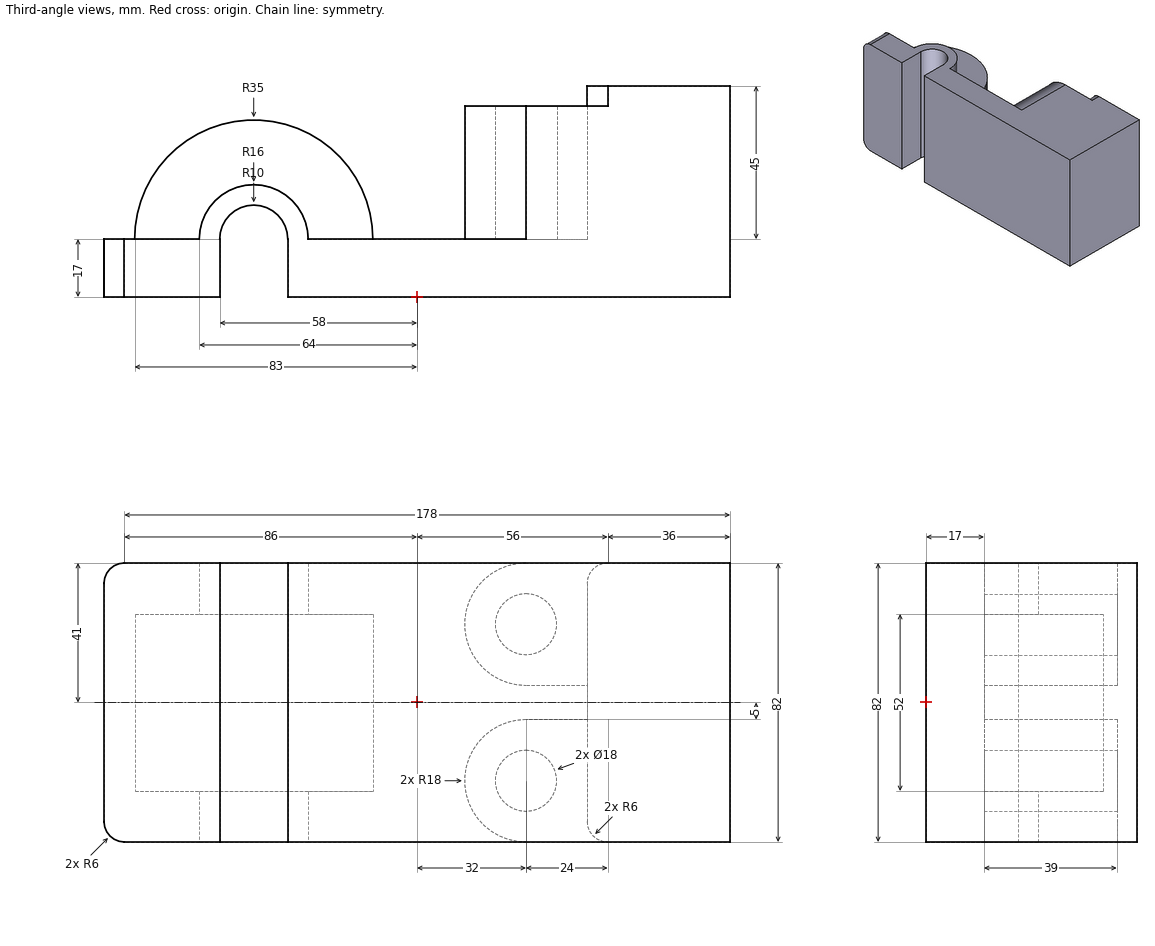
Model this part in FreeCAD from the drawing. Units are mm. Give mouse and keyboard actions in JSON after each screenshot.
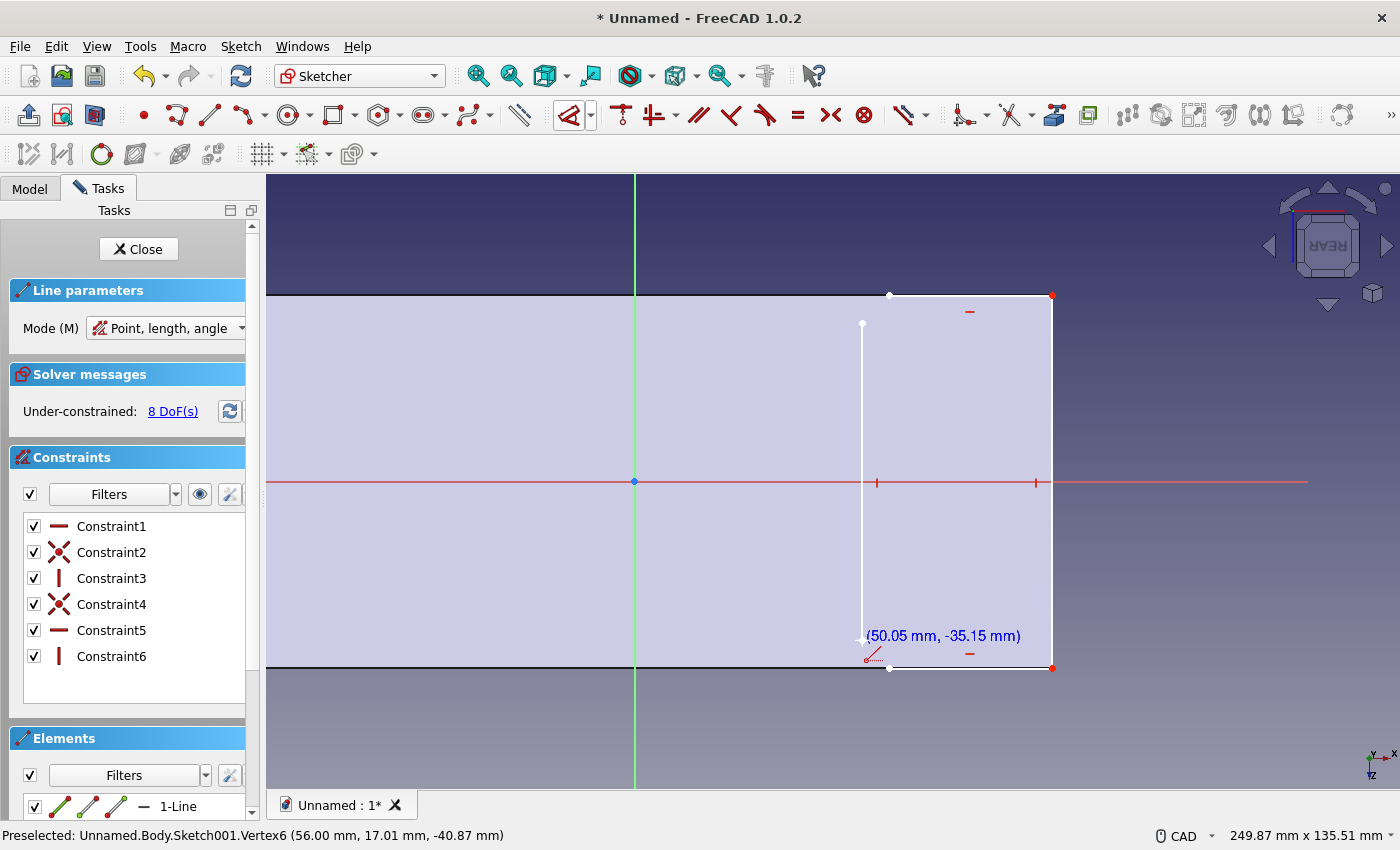
{"action": "left_click", "coordinate": [242, 116]}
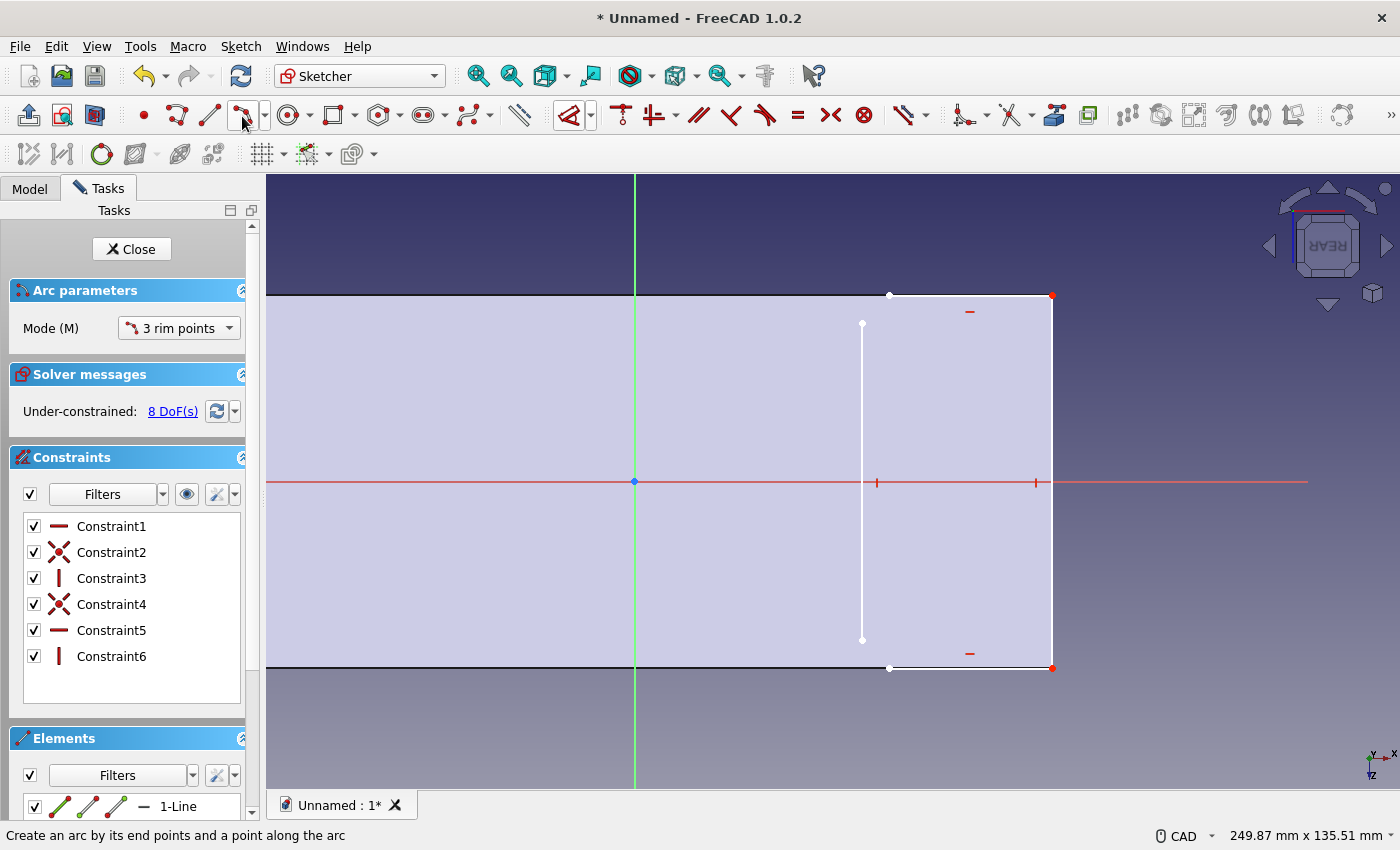
{"action": "left_click", "coordinate": [889, 296]}
{"action": "left_click", "coordinate": [862, 324]}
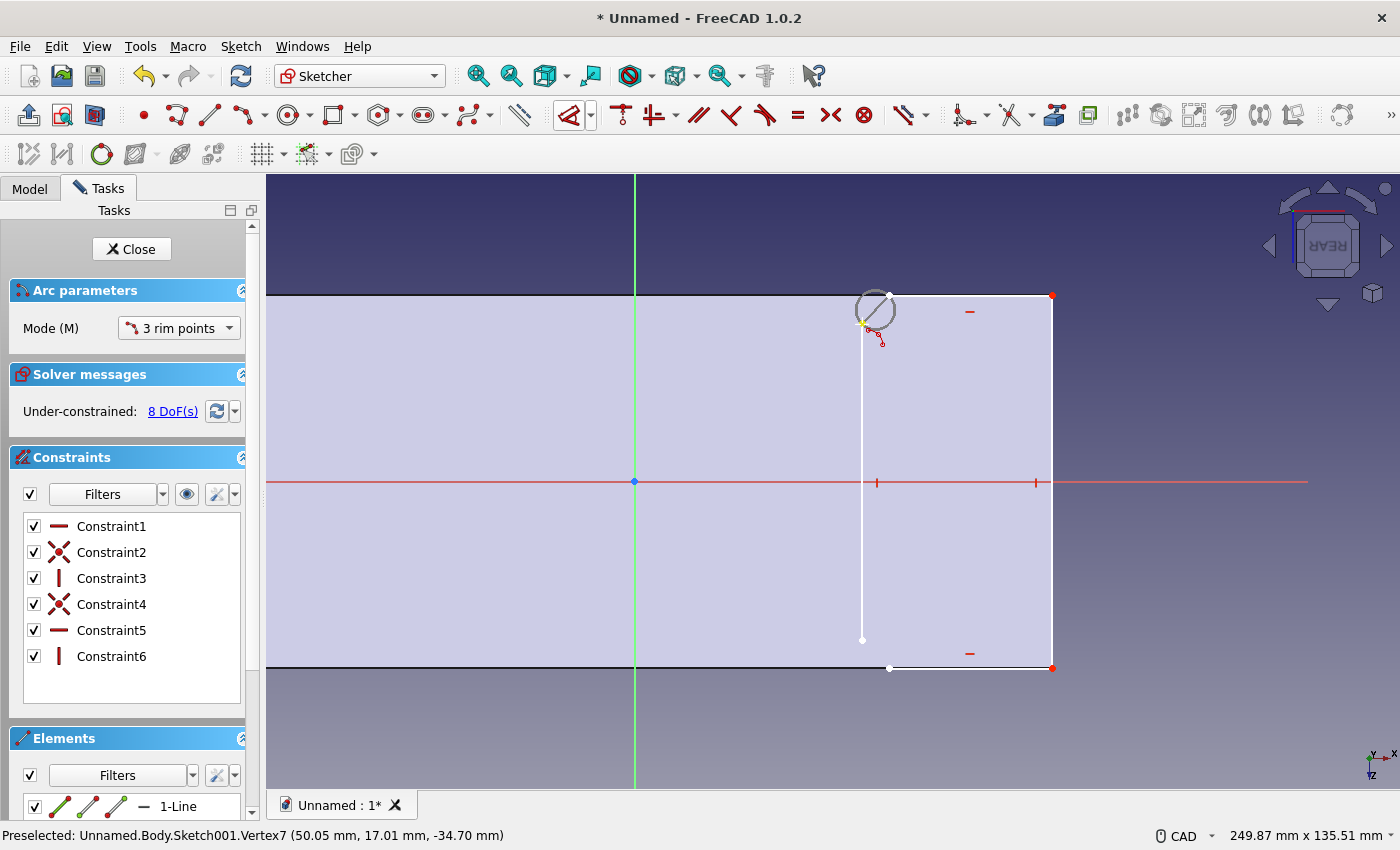
{"action": "scroll", "coordinate": [870, 303], "scroll_direction": "up", "scroll_amount": 4}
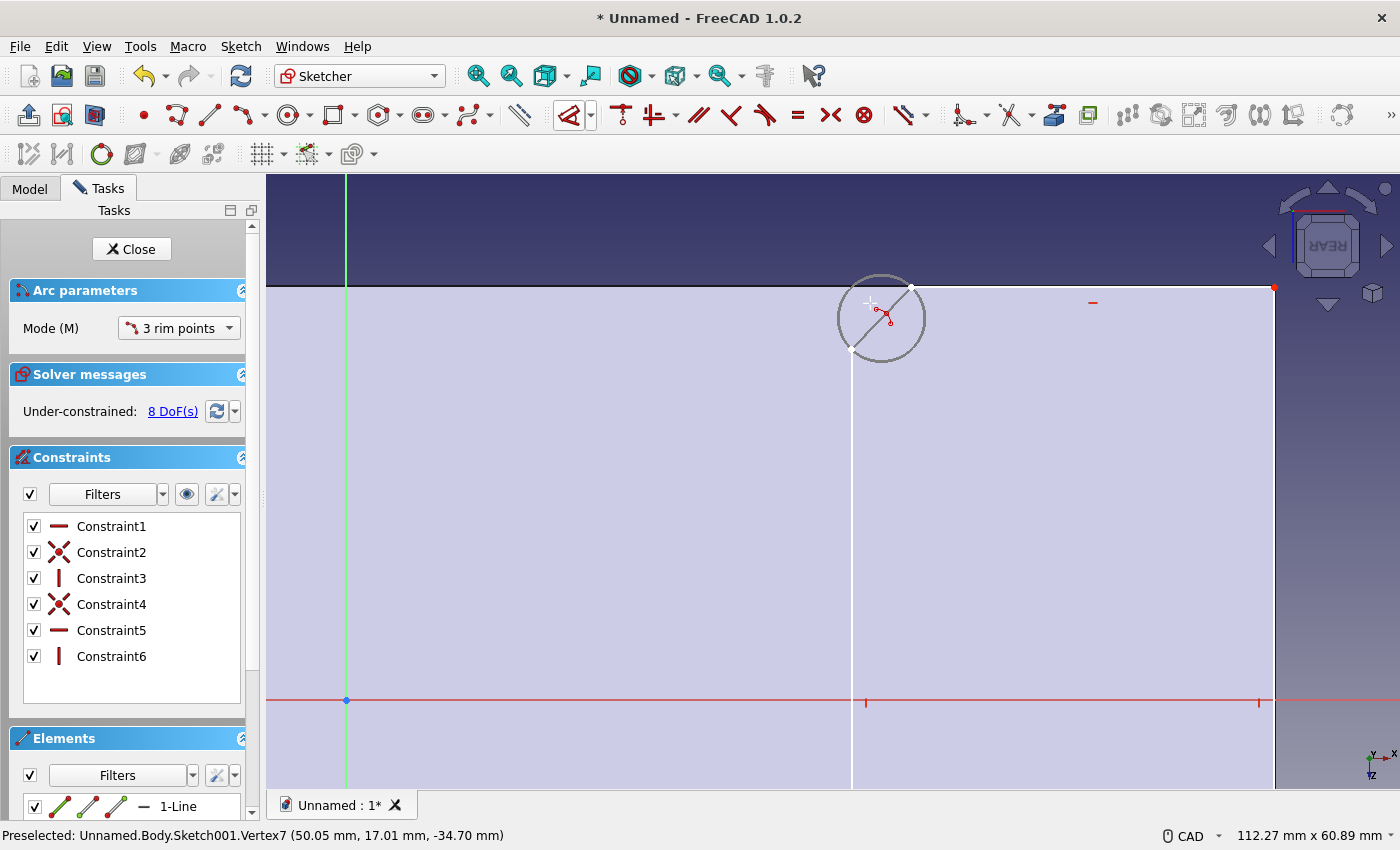
{"action": "left_click", "coordinate": [869, 304]}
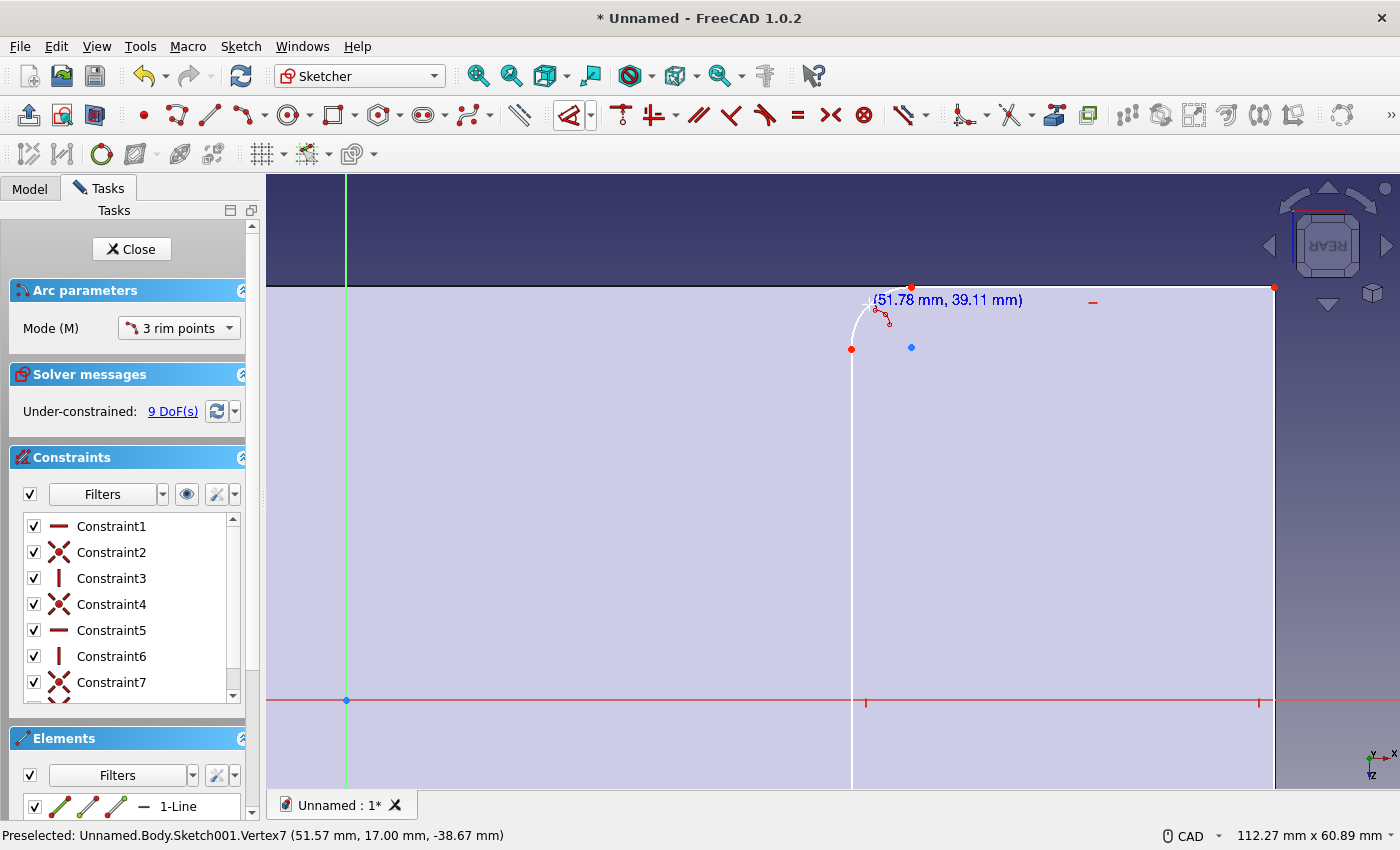
{"action": "scroll", "coordinate": [727, 303], "scroll_direction": "down", "scroll_amount": 4}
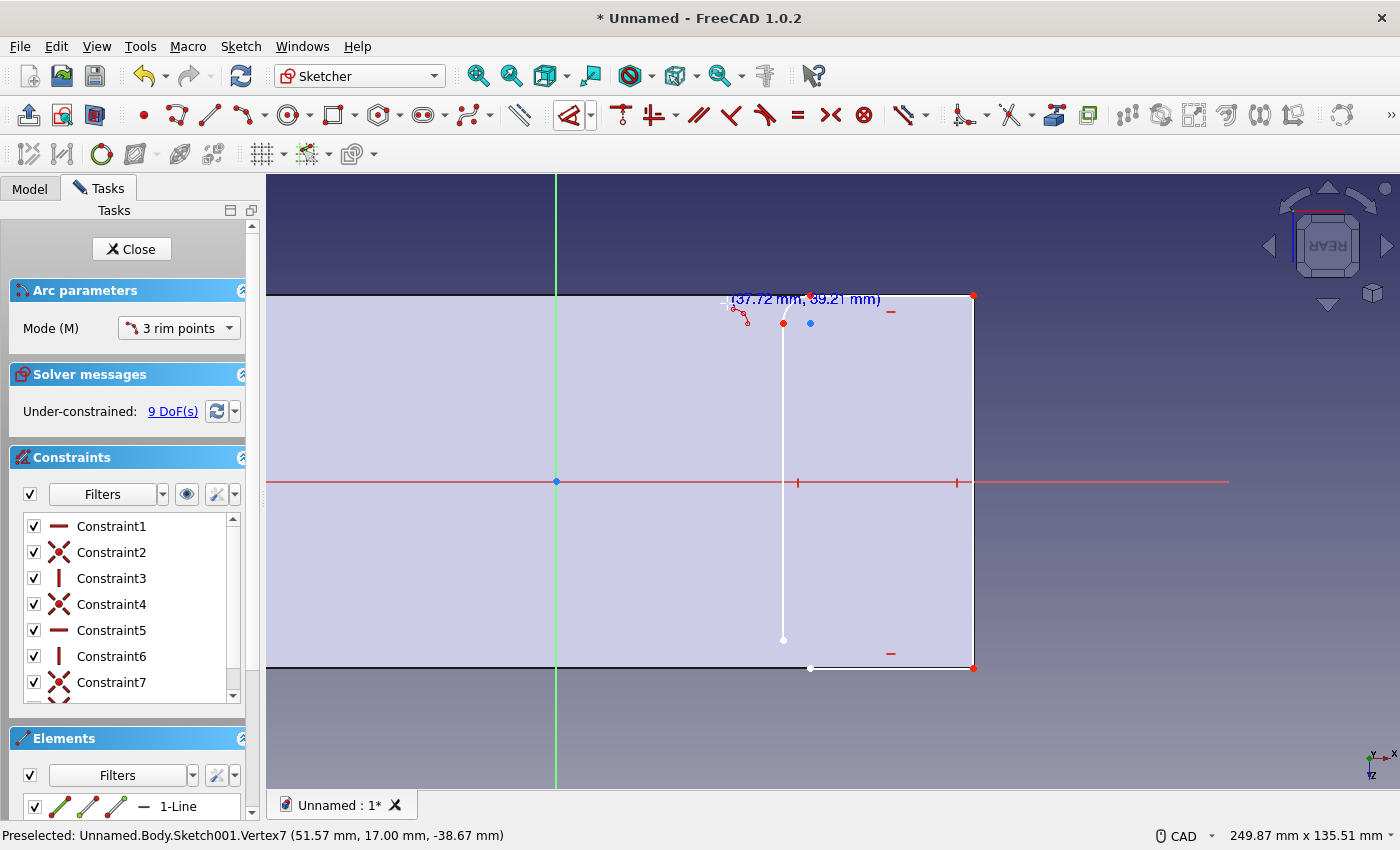
{"action": "left_click", "coordinate": [783, 641]}
{"action": "left_click", "coordinate": [810, 669]}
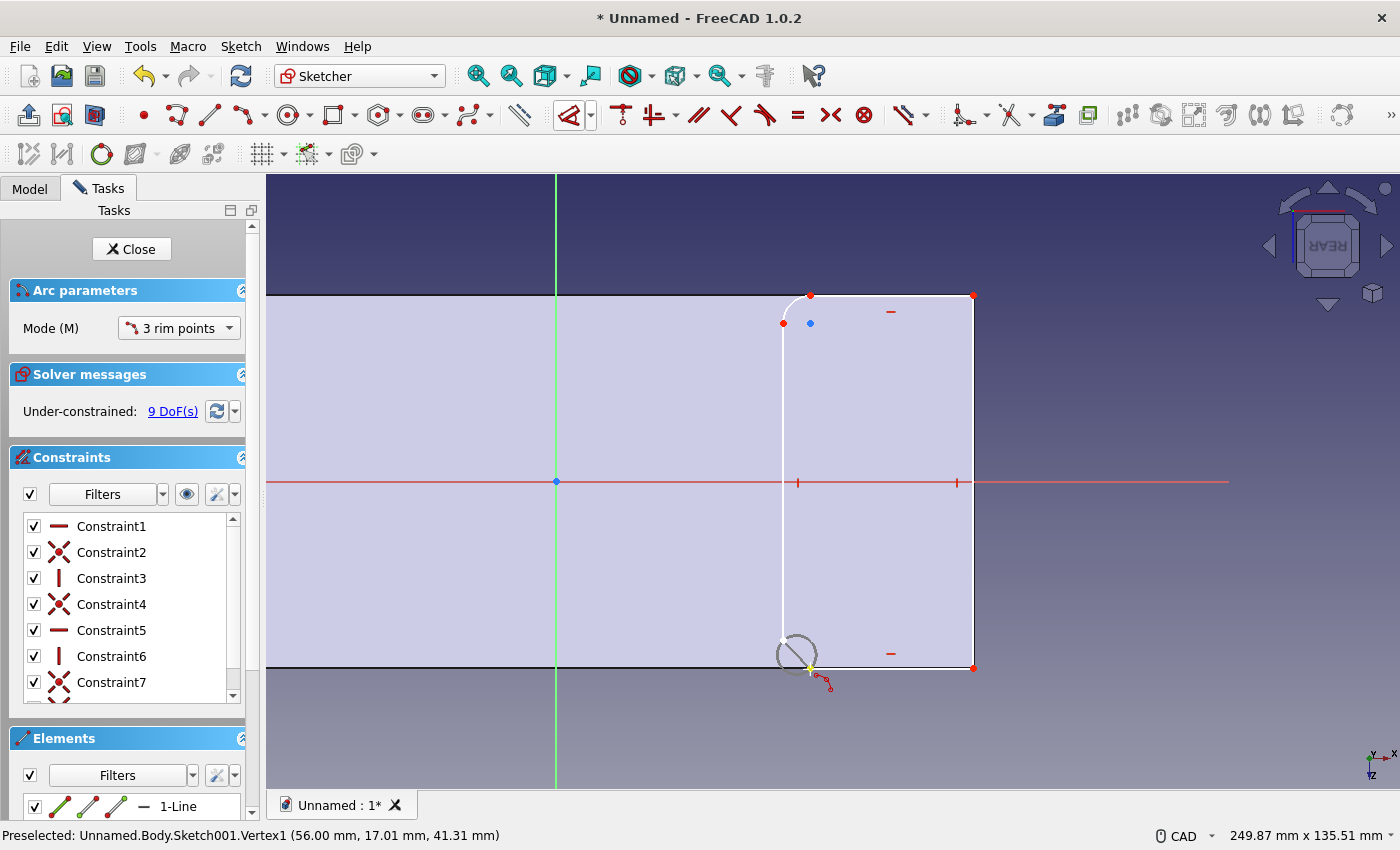
{"action": "scroll", "coordinate": [791, 660], "scroll_direction": "up", "scroll_amount": 4}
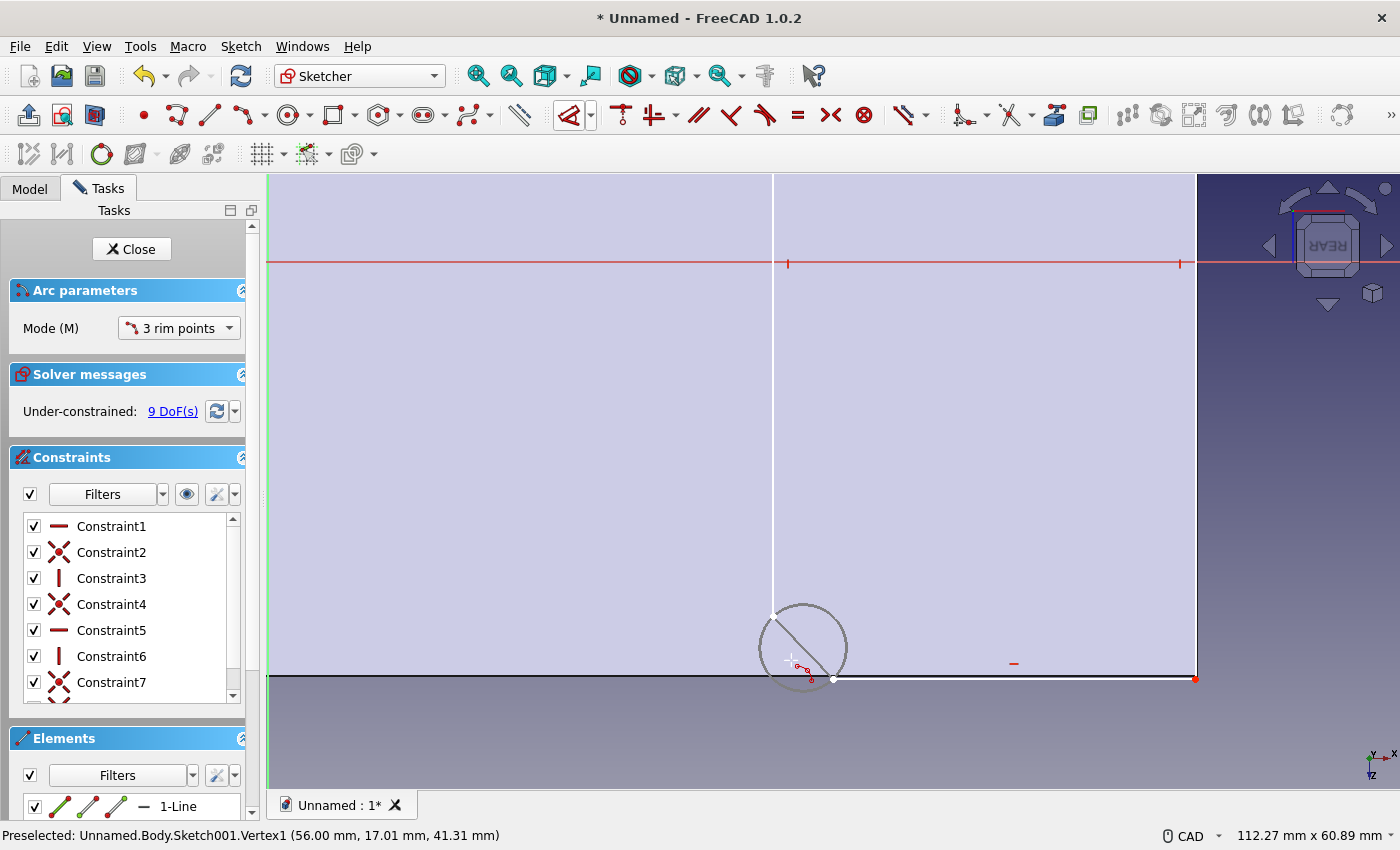
{"action": "left_click", "coordinate": [790, 658]}
{"action": "key", "text": "Escape"}